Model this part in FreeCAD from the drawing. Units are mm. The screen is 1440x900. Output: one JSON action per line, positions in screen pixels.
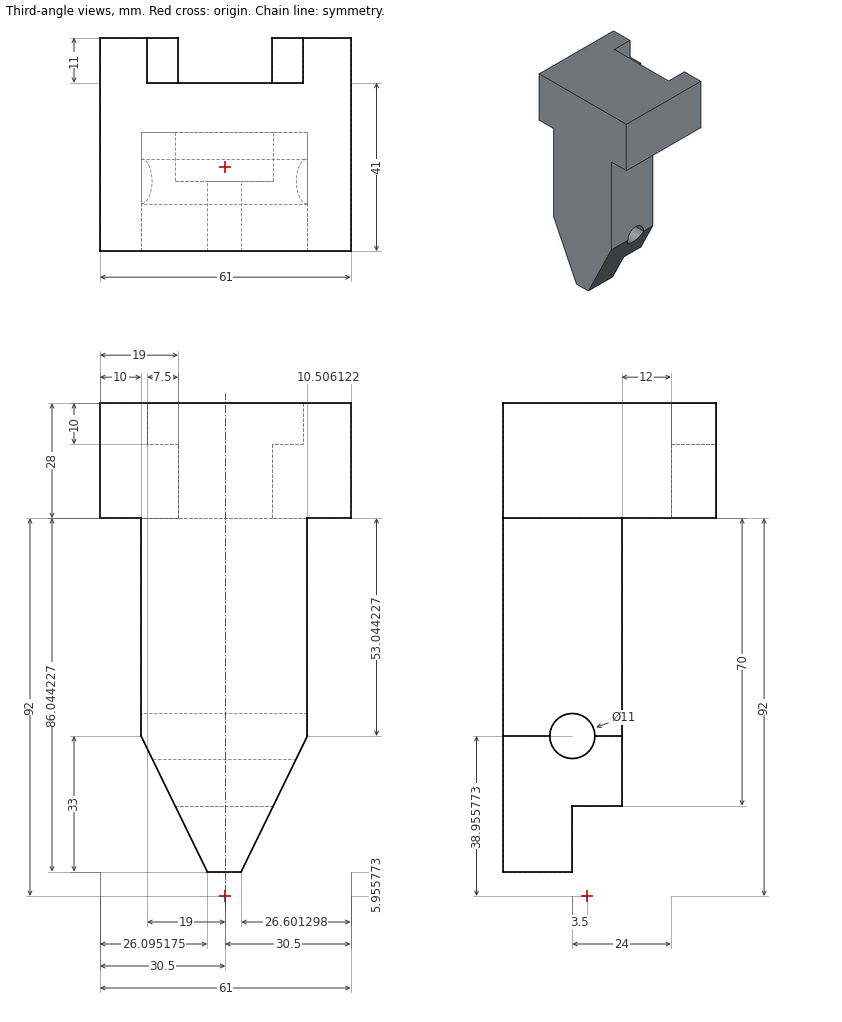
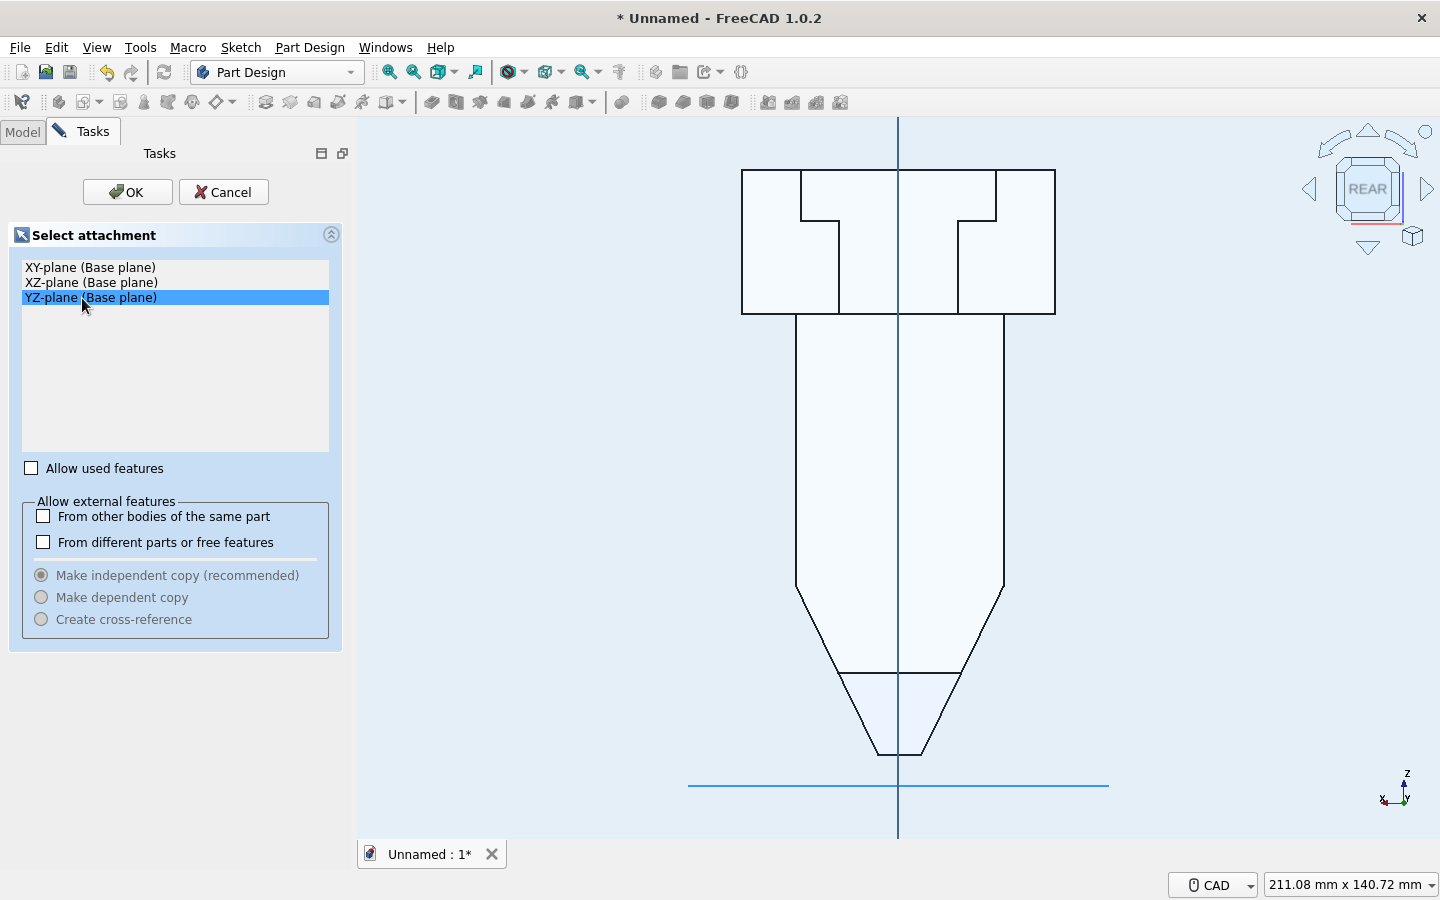
{"action": "left_click", "coordinate": [128, 192]}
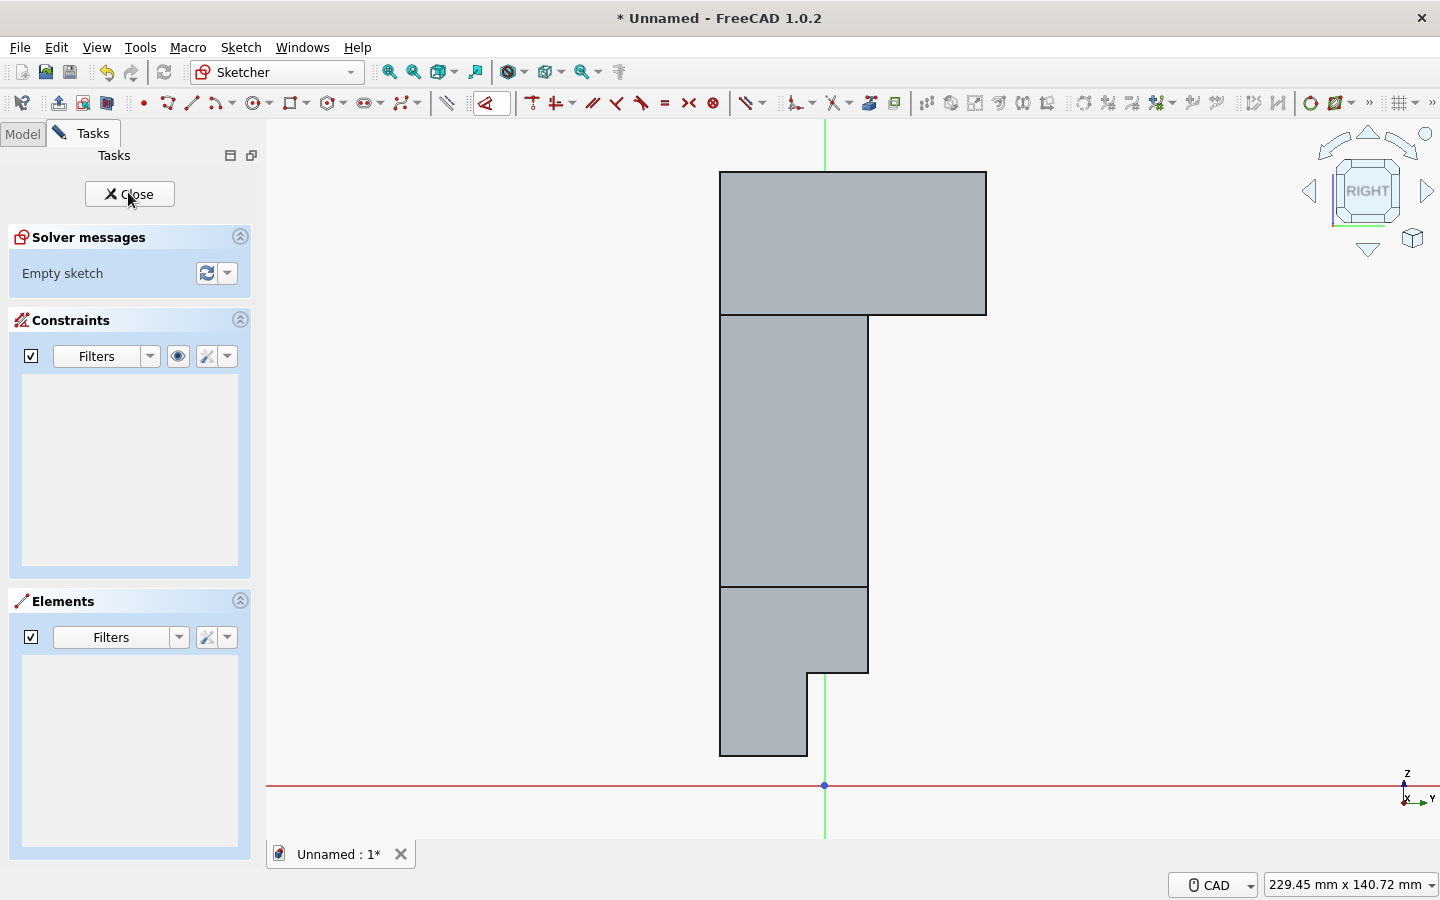
{"action": "left_click", "coordinate": [108, 104]}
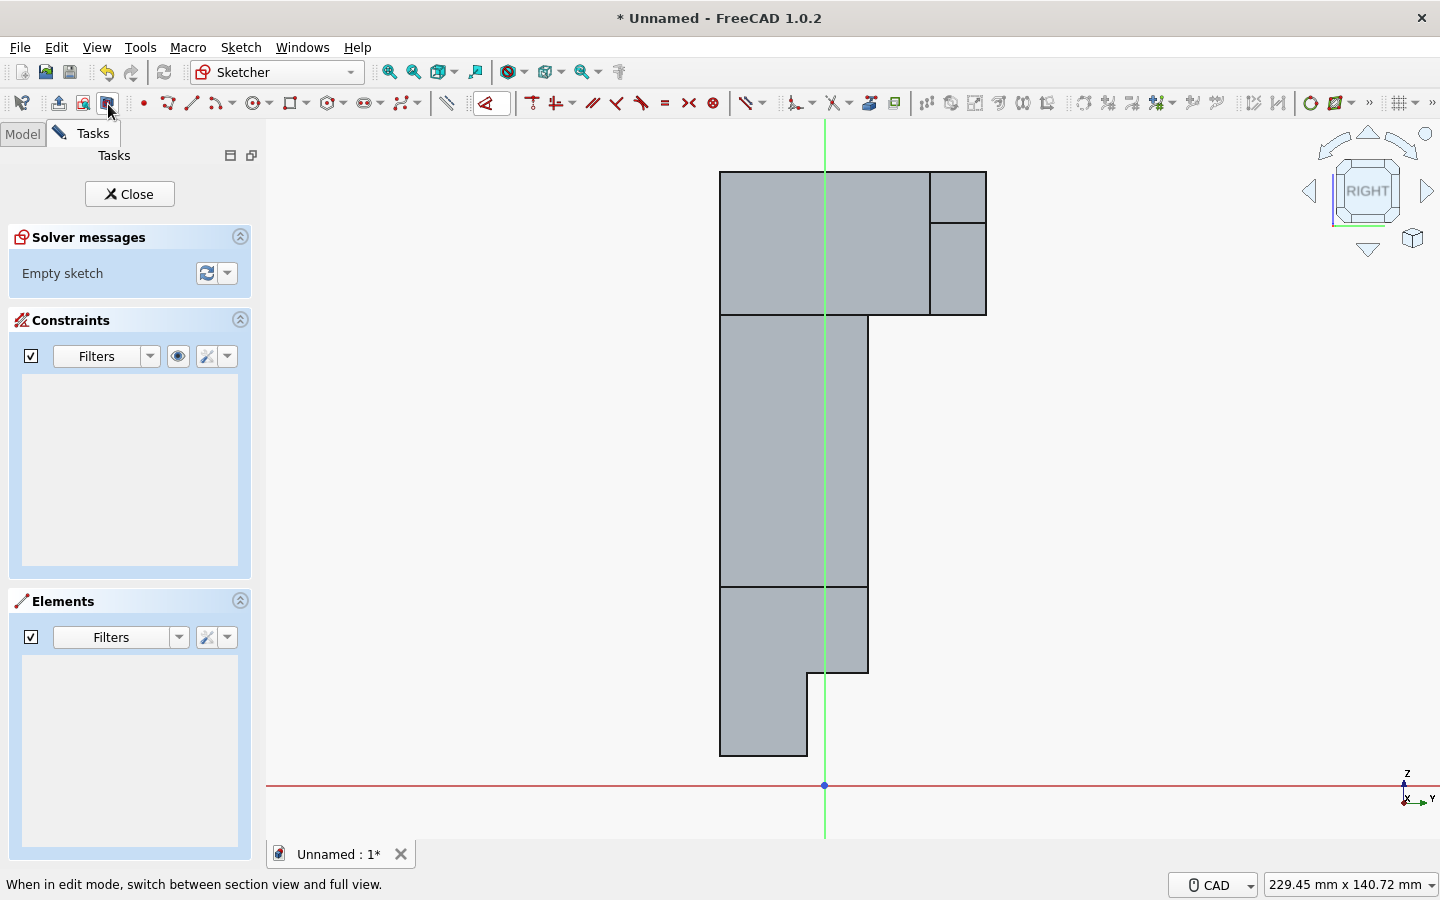
{"action": "scroll", "coordinate": [810, 600], "scroll_direction": "up", "scroll_amount": 11}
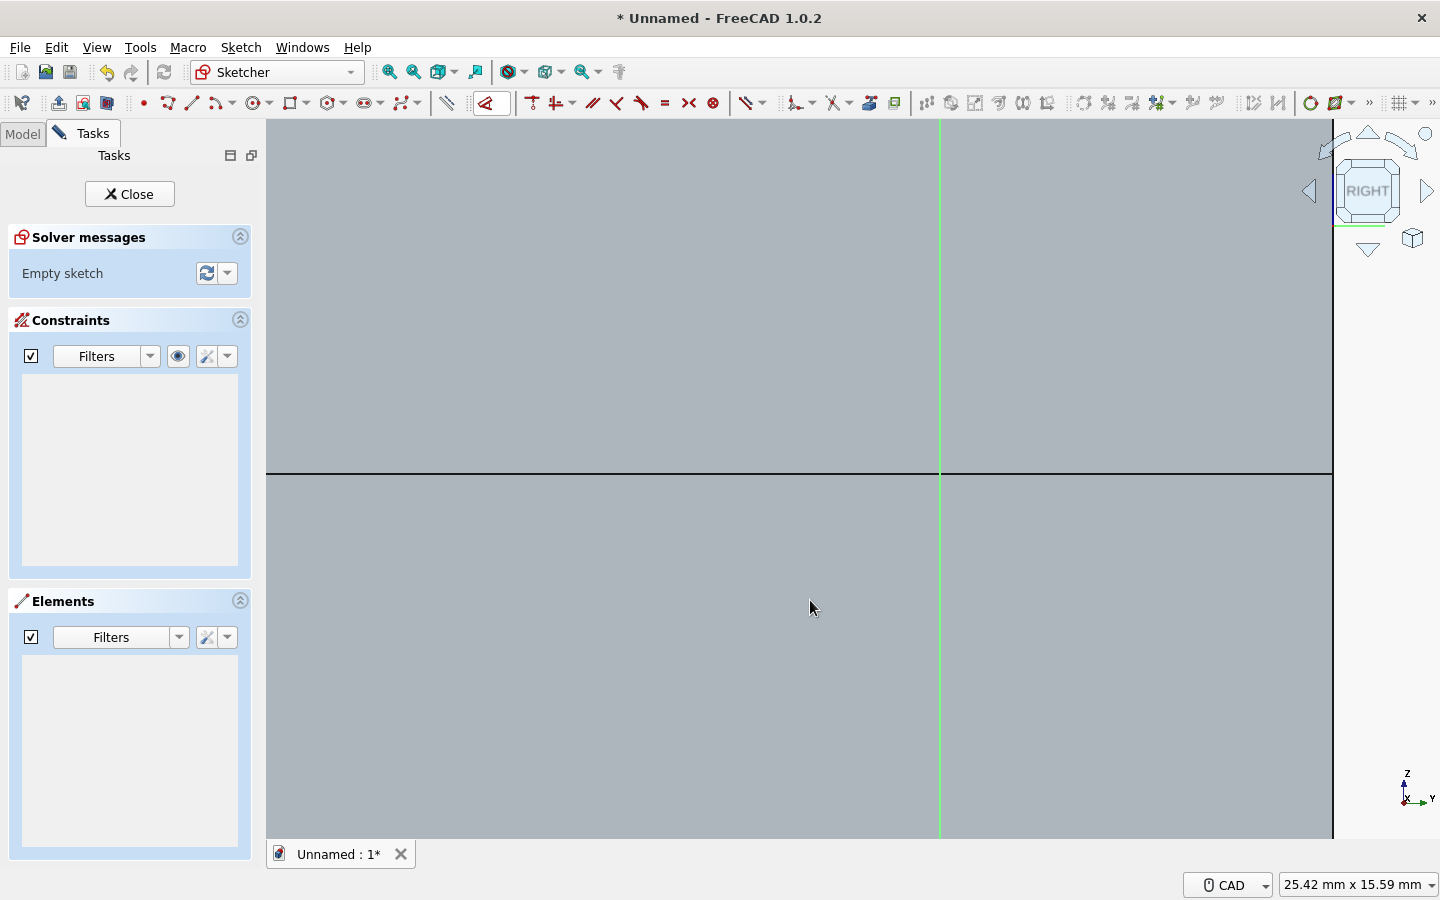
{"action": "left_click", "coordinate": [254, 104]}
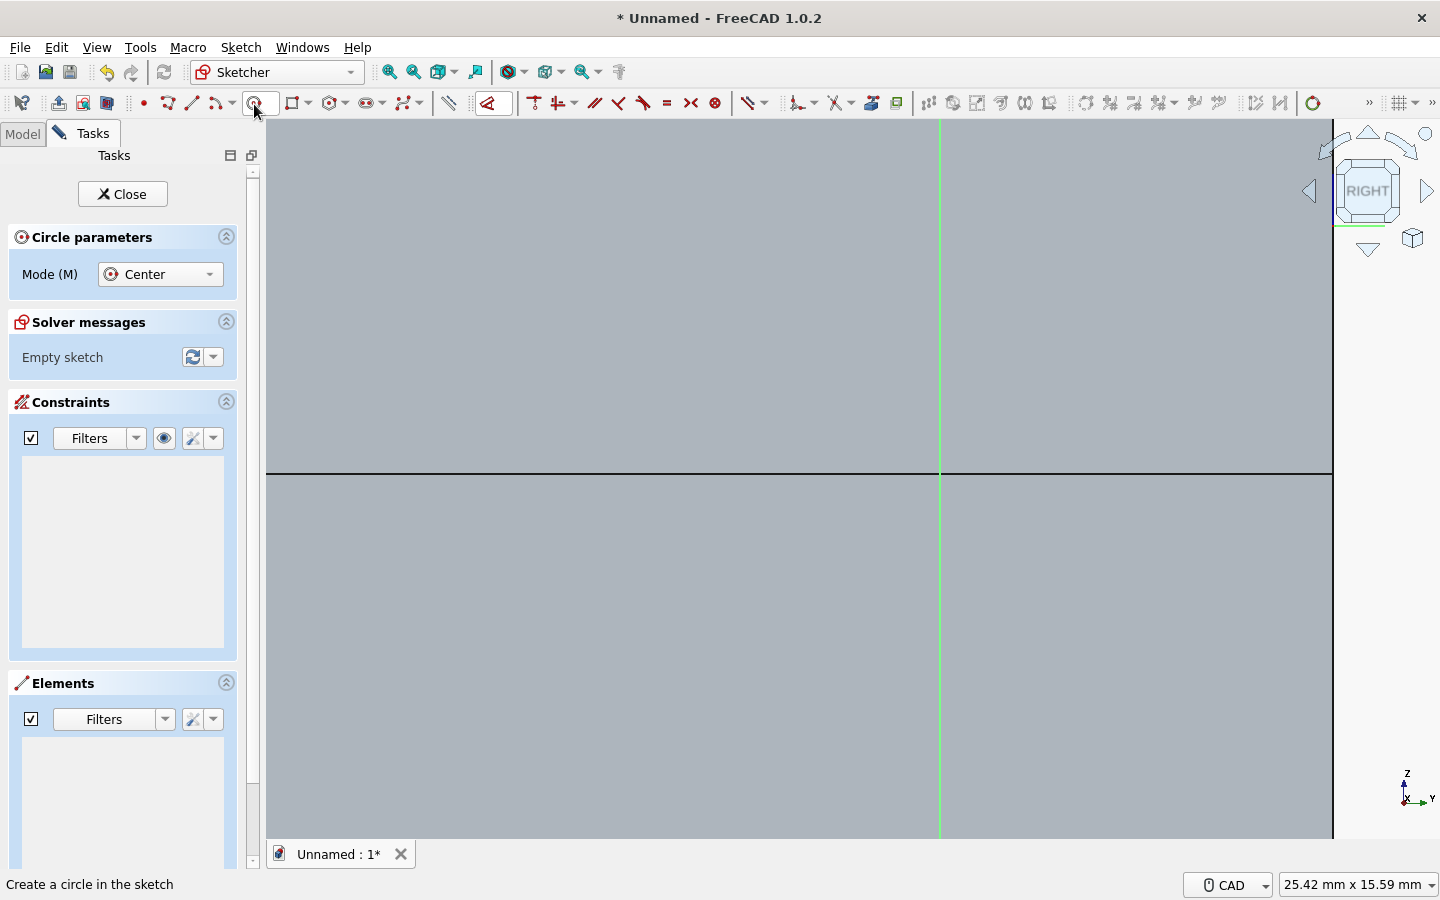
{"action": "left_click", "coordinate": [779, 474]}
{"action": "left_click", "coordinate": [958, 295]}
{"action": "key", "text": "Escape"}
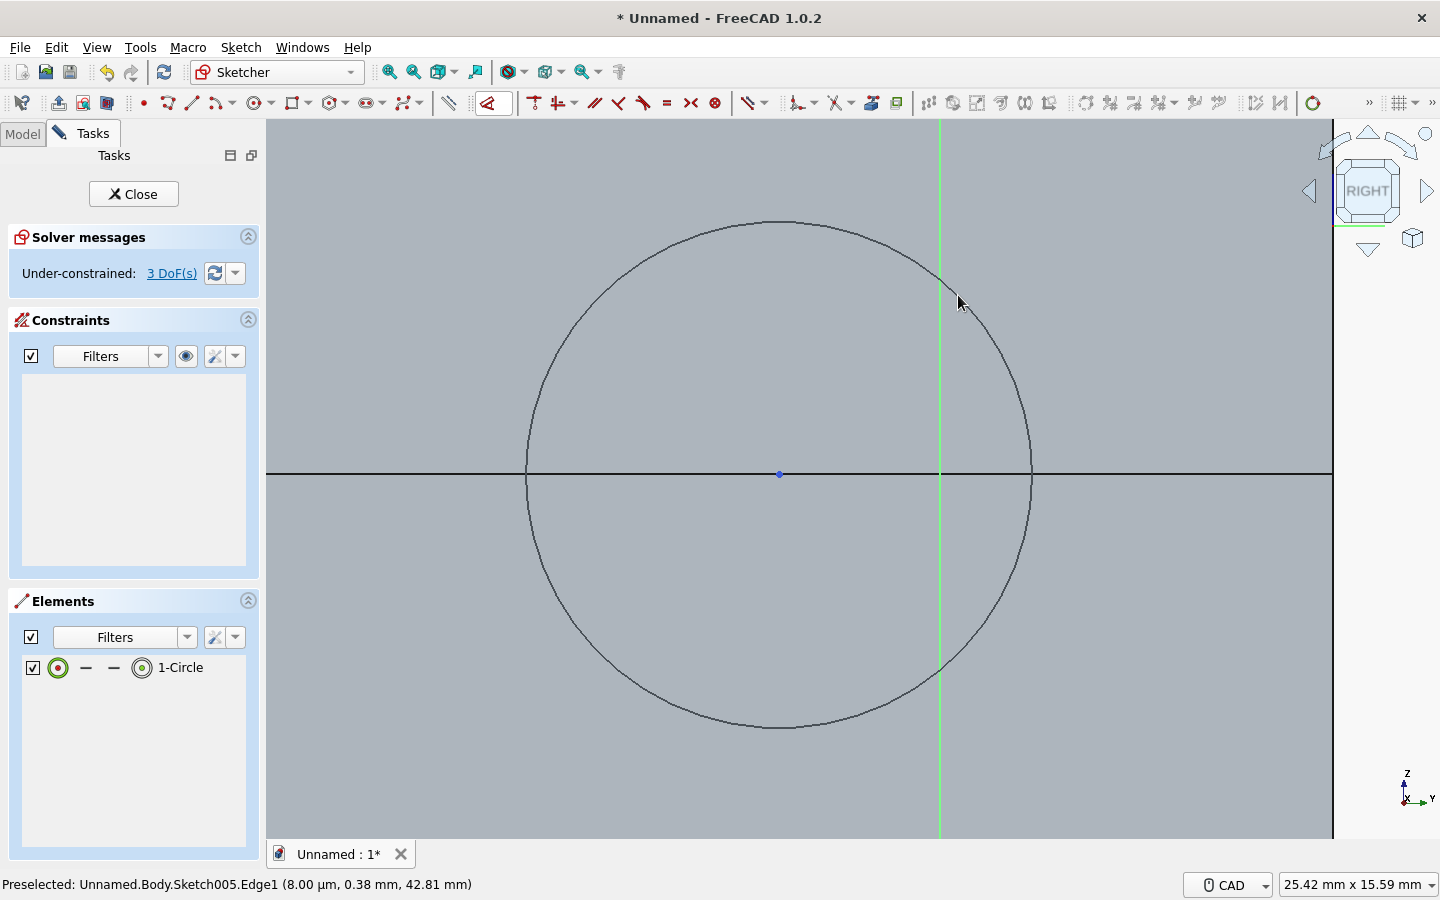
{"action": "left_click", "coordinate": [957, 295]}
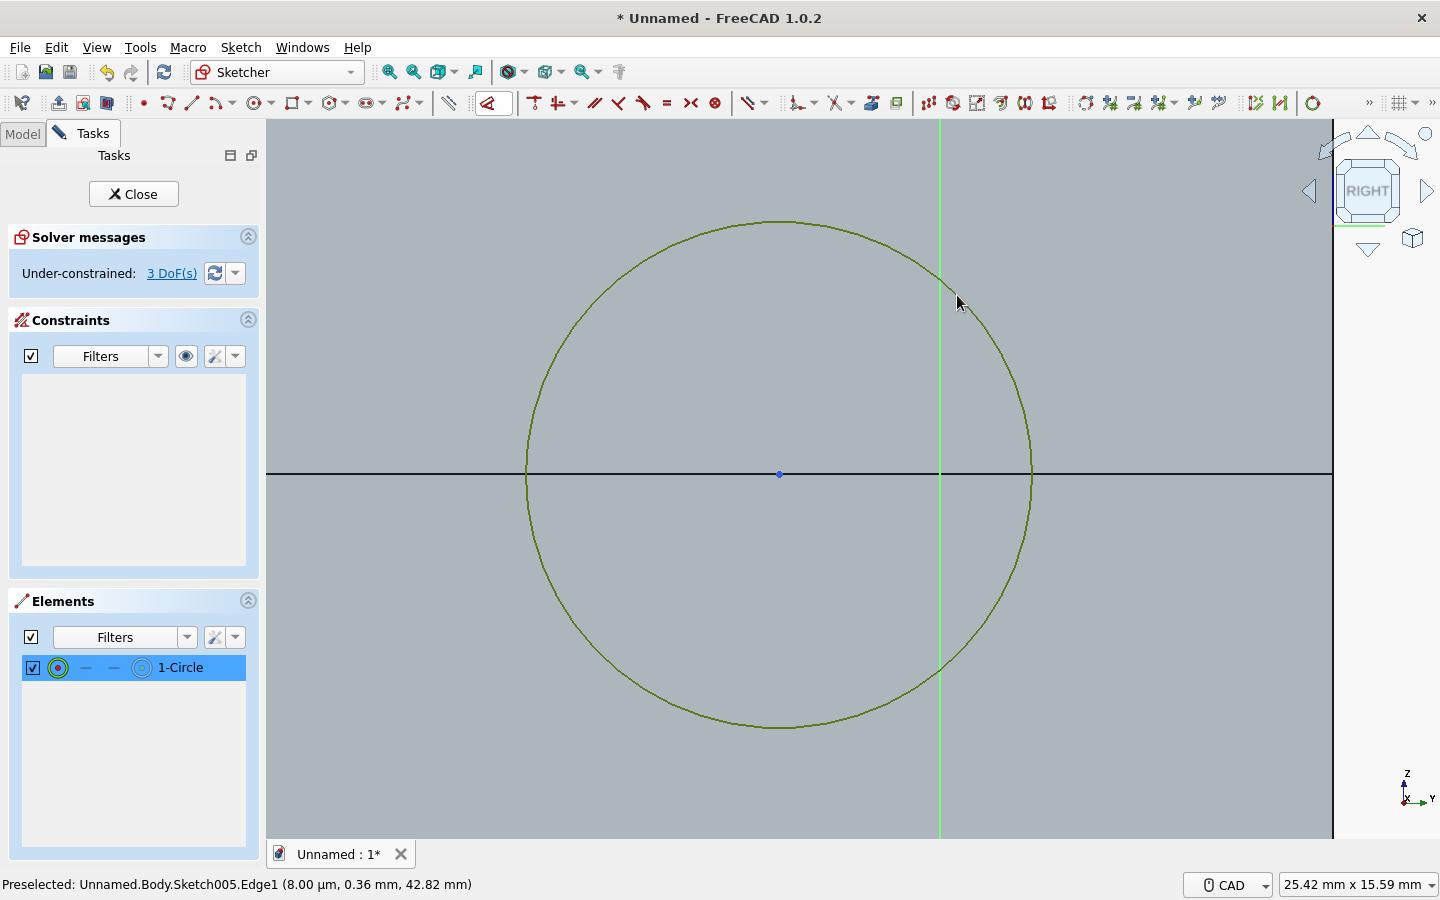
{"action": "left_click", "coordinate": [506, 104]}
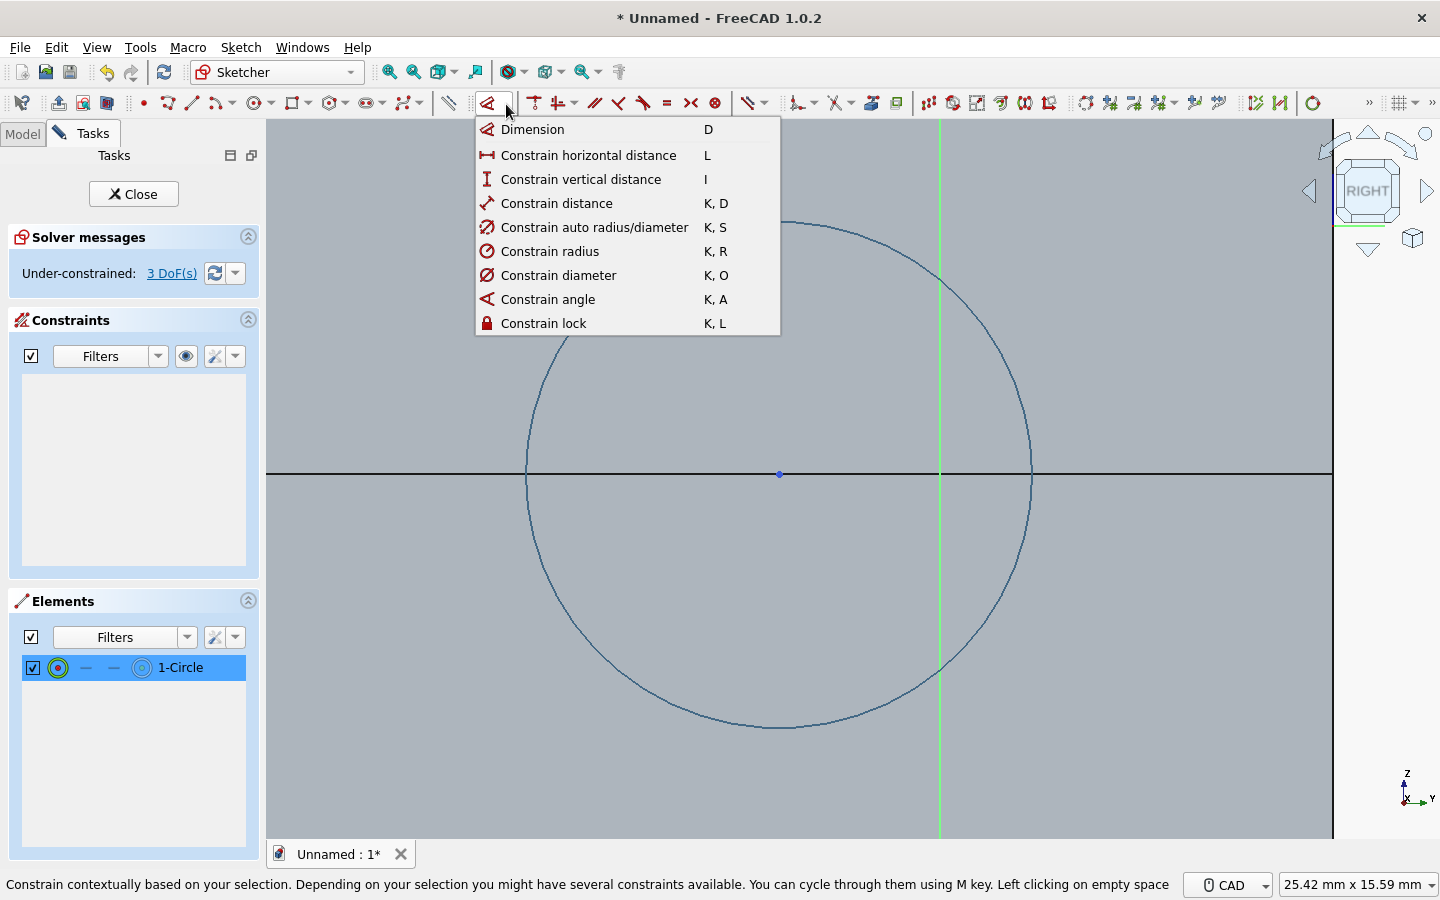
{"action": "left_click", "coordinate": [628, 275]}